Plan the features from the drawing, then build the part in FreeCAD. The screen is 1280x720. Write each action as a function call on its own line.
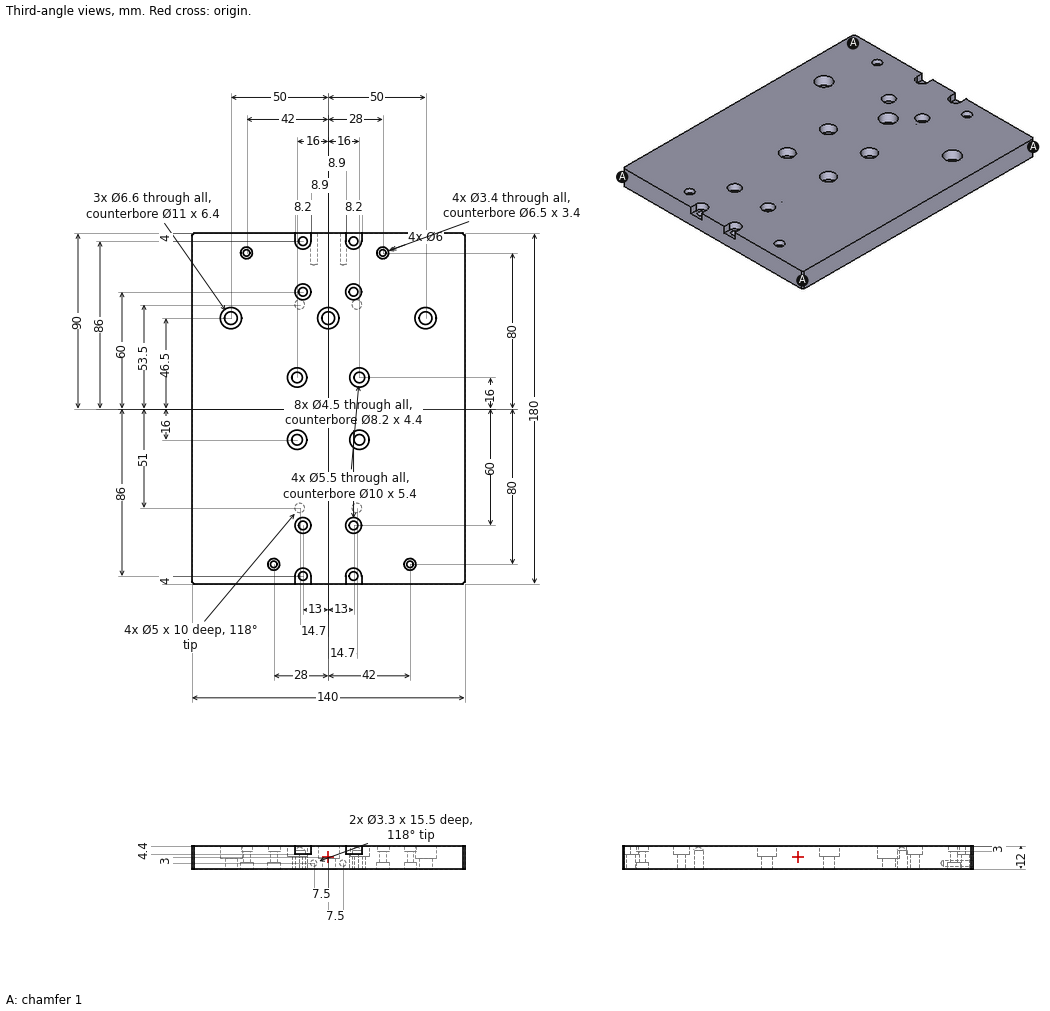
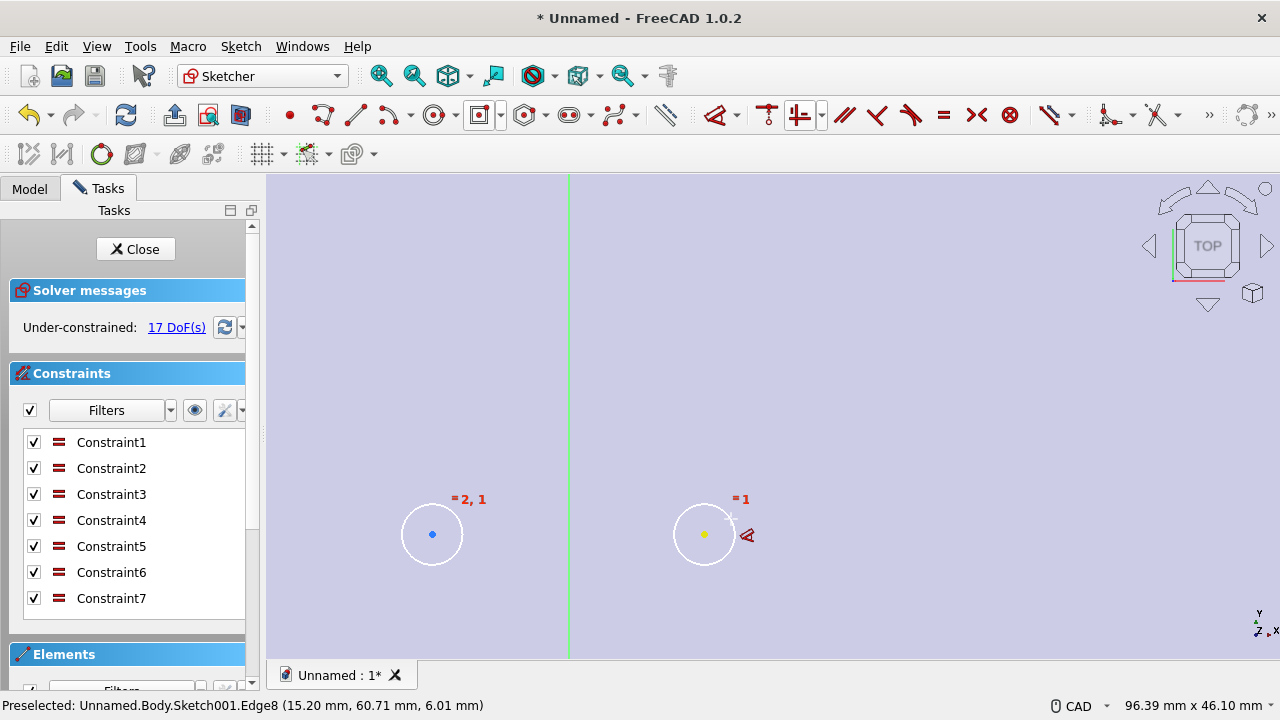
click(726, 513)
click(749, 490)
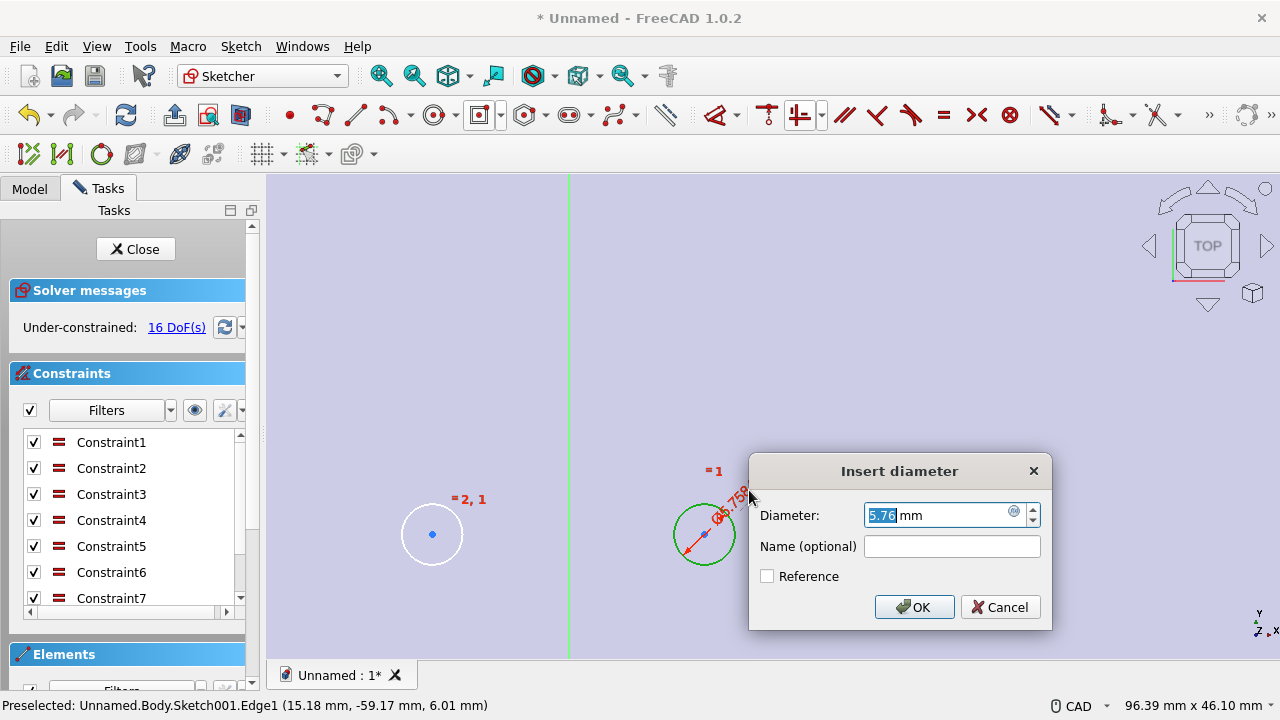
text(4.5)
key(Return)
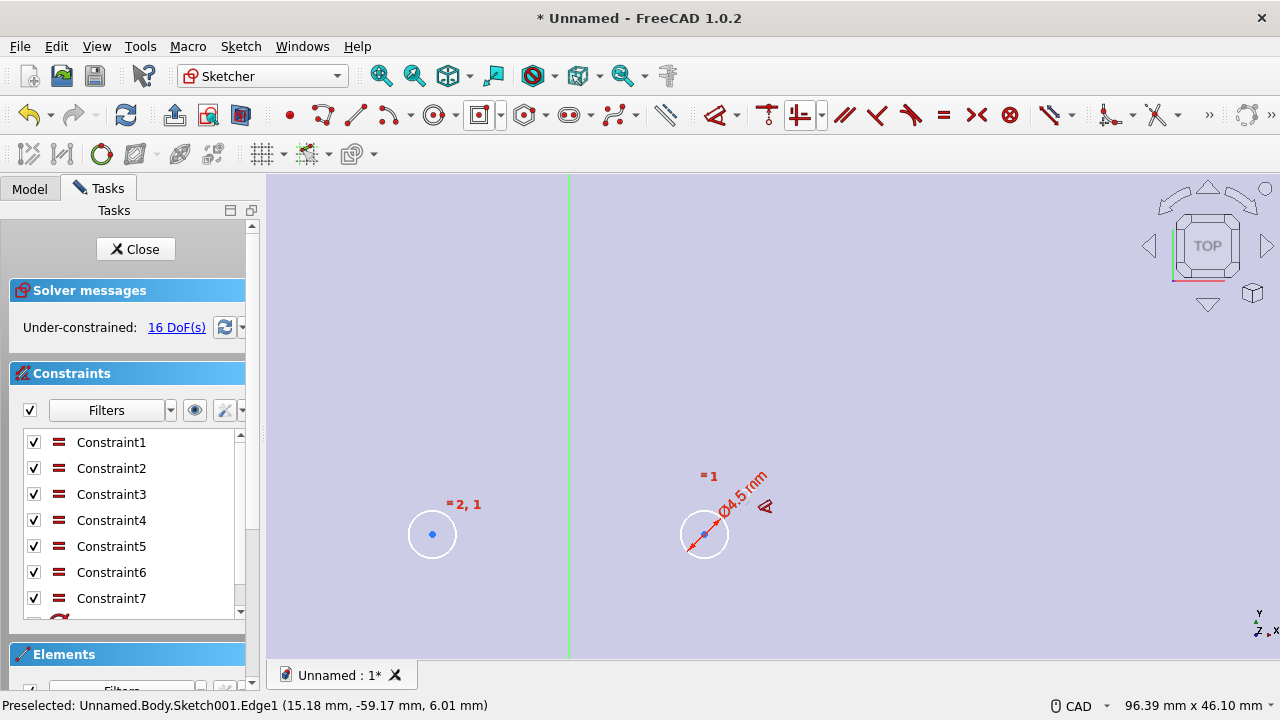
scroll(731, 520, down, 9)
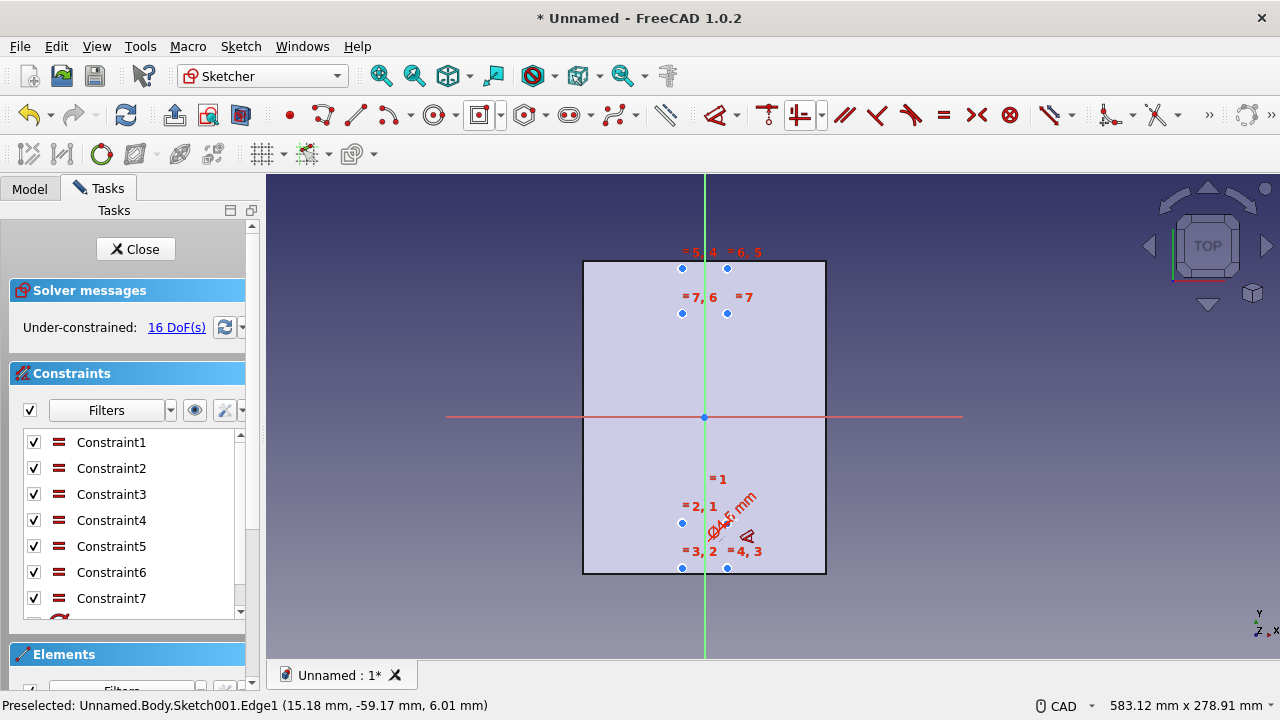
scroll(727, 523, up, 3)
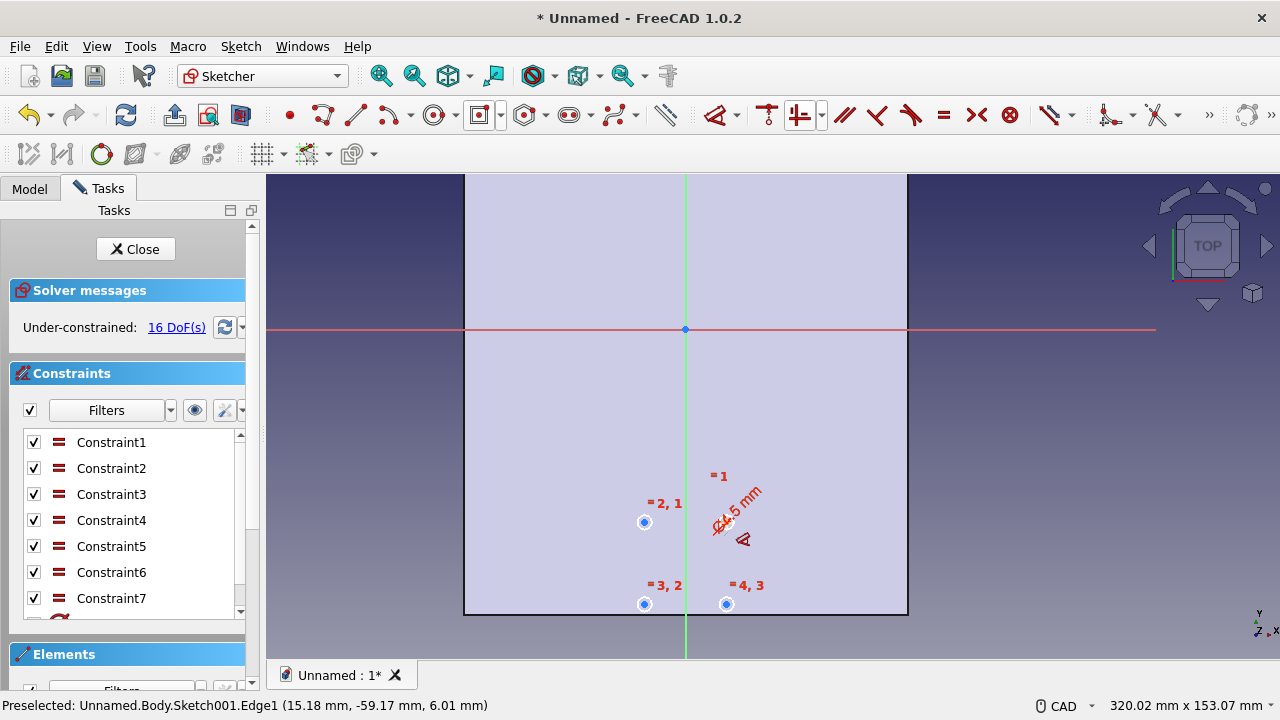
click(727, 522)
click(706, 556)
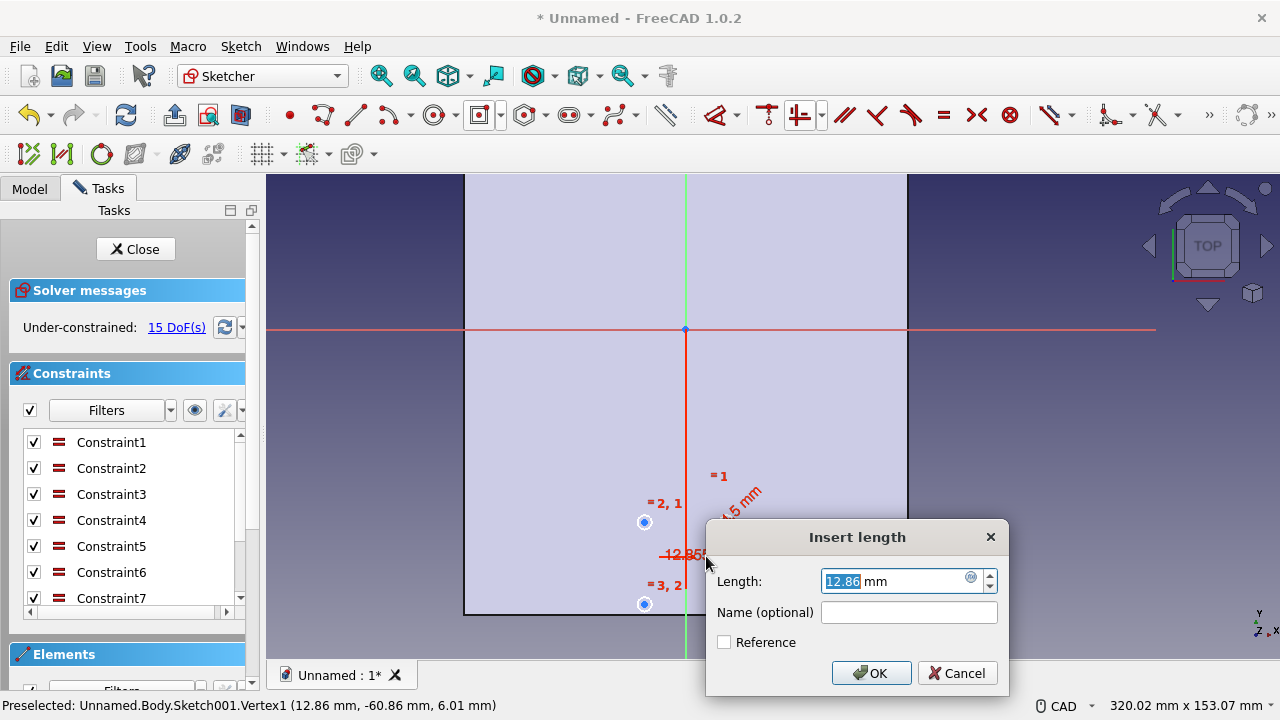
text(13)
key(Return)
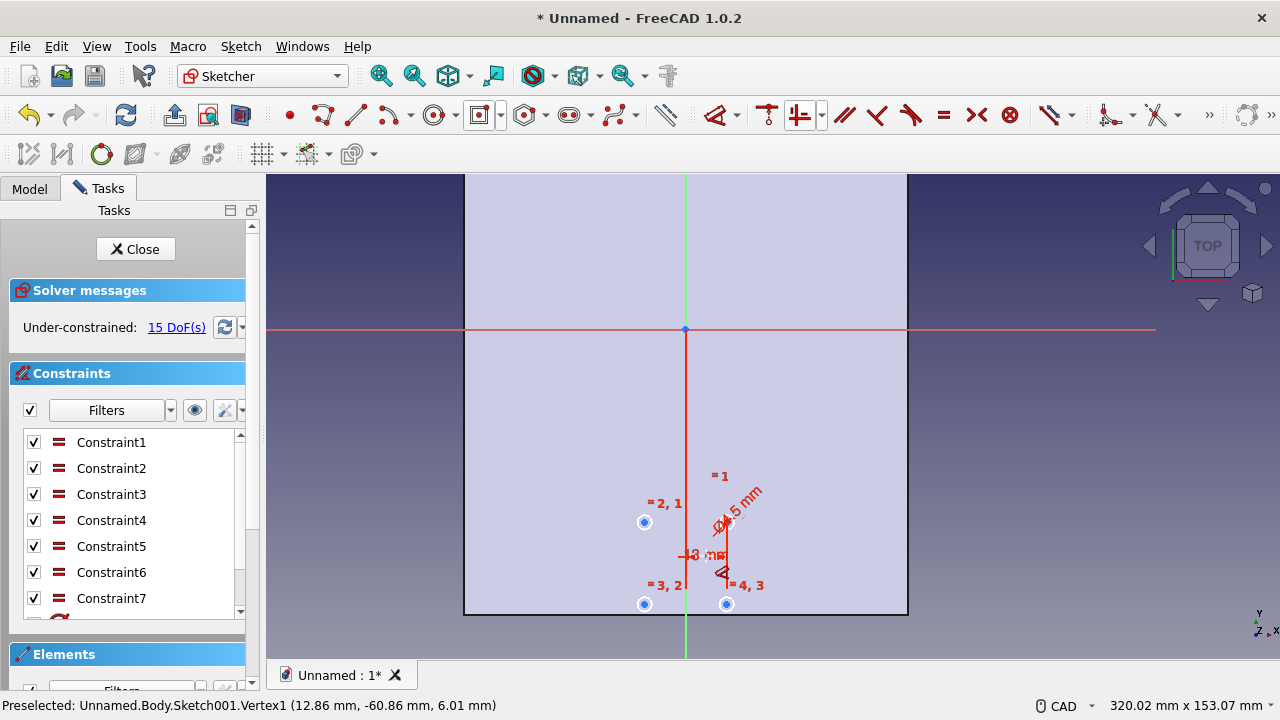
click(727, 522)
click(761, 426)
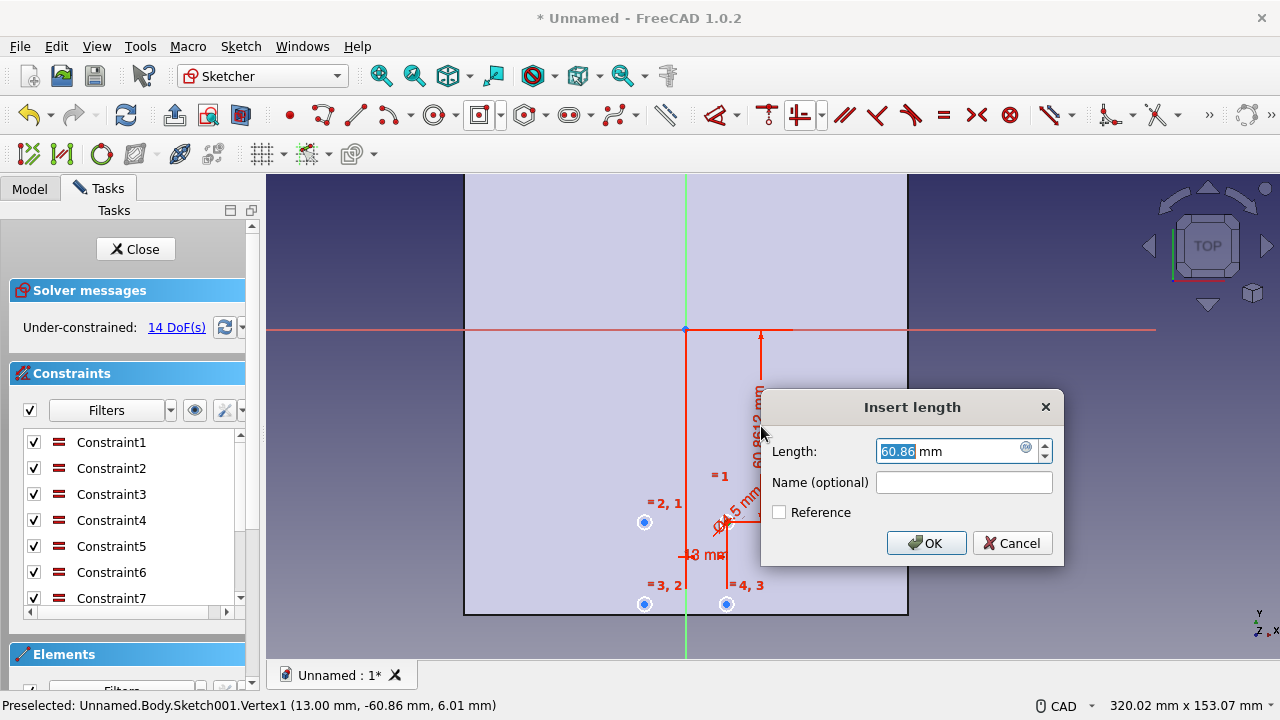
text(60)
key(Return)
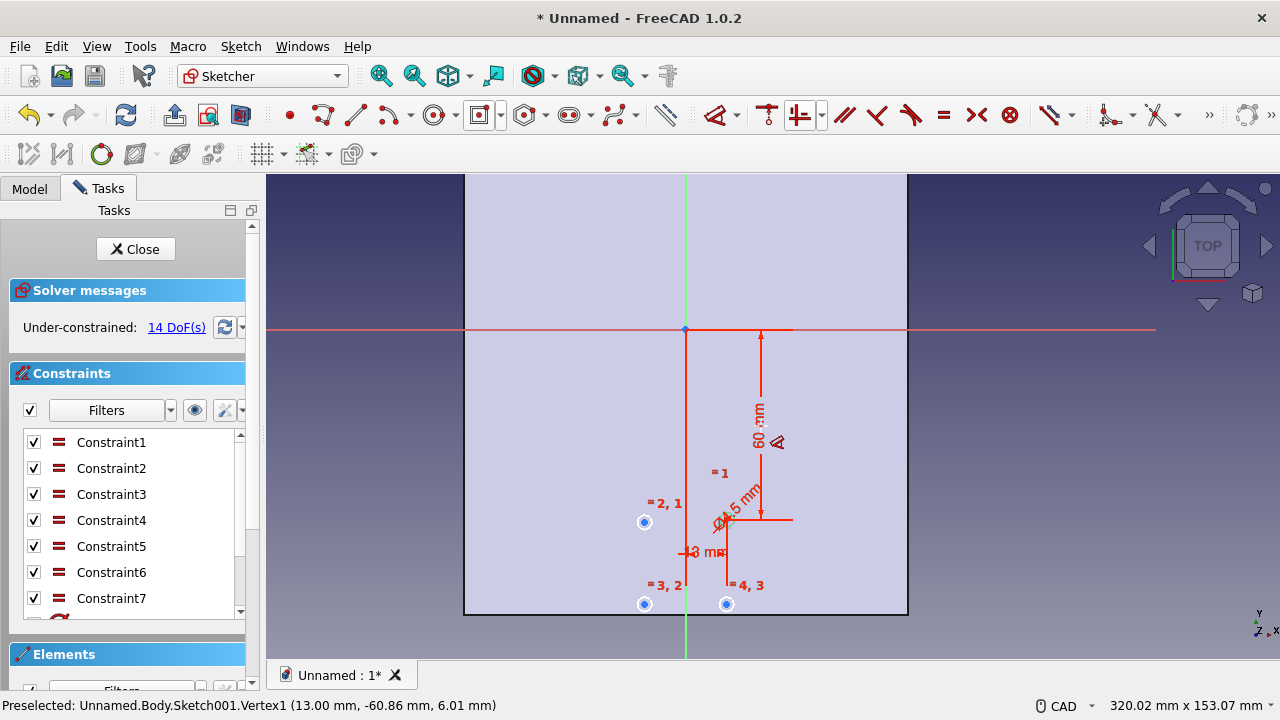
click(645, 522)
click(665, 296)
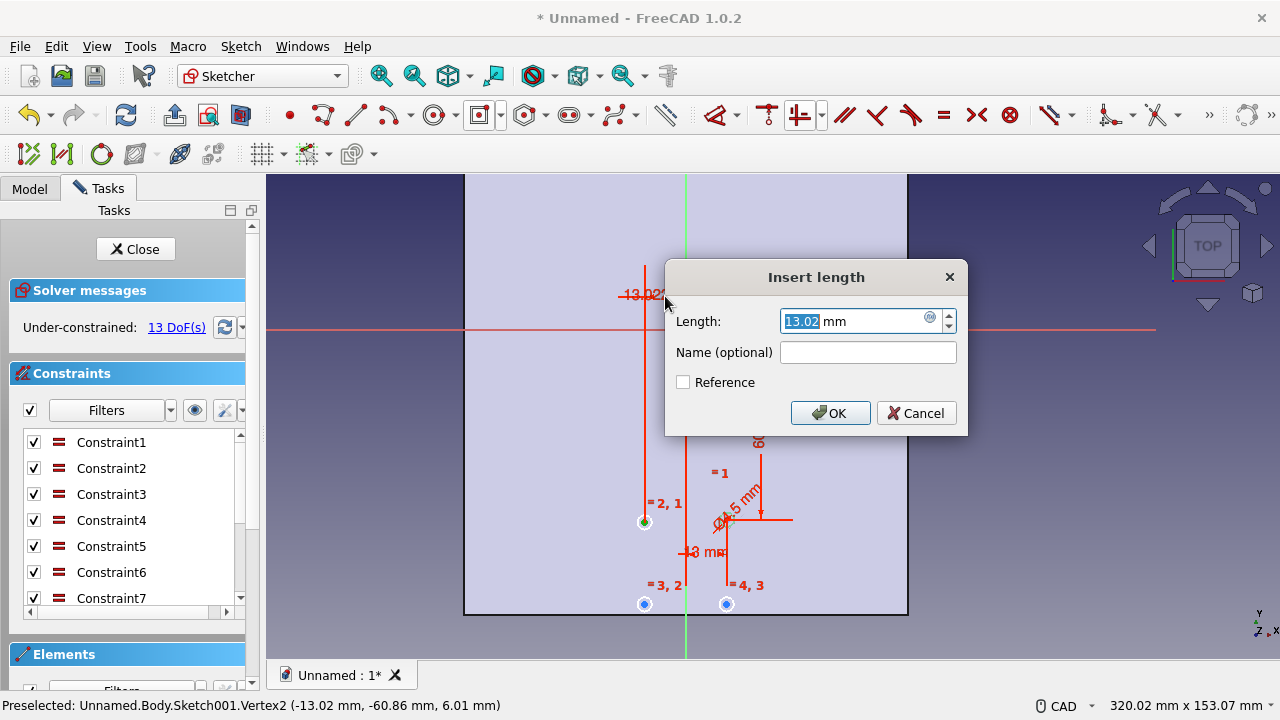
text(13)
key(Return)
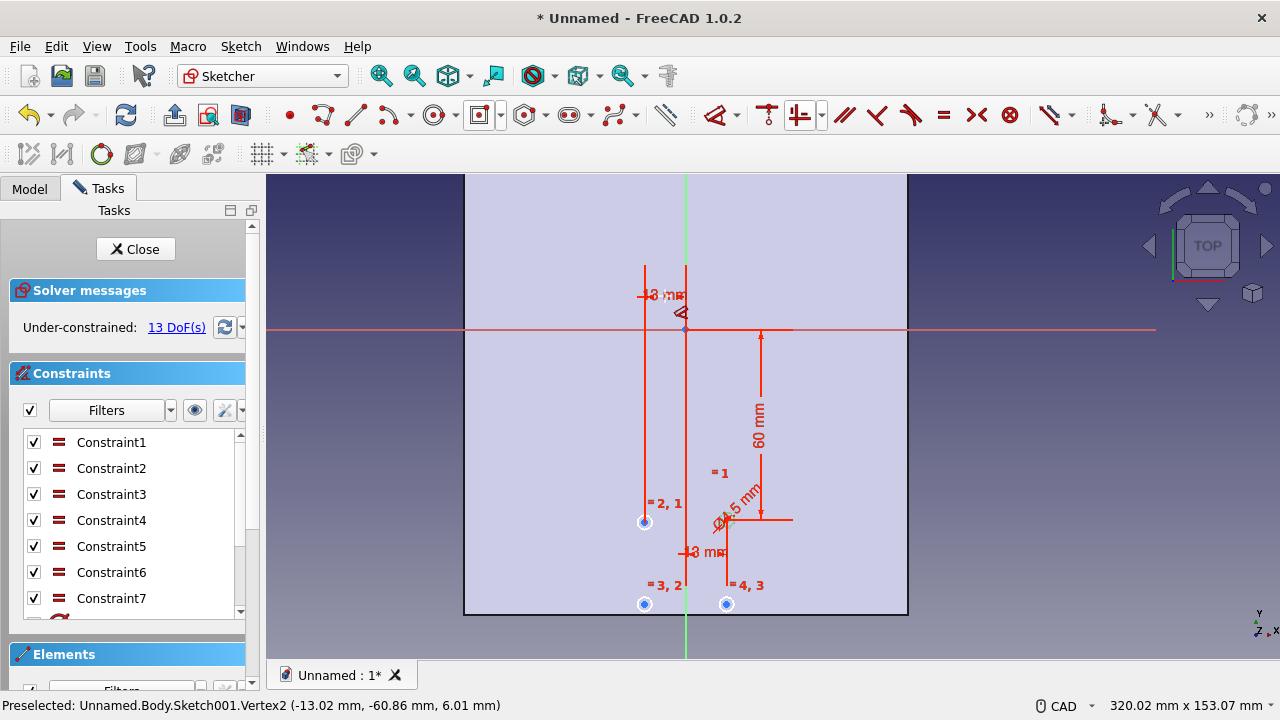
click(645, 522)
click(611, 426)